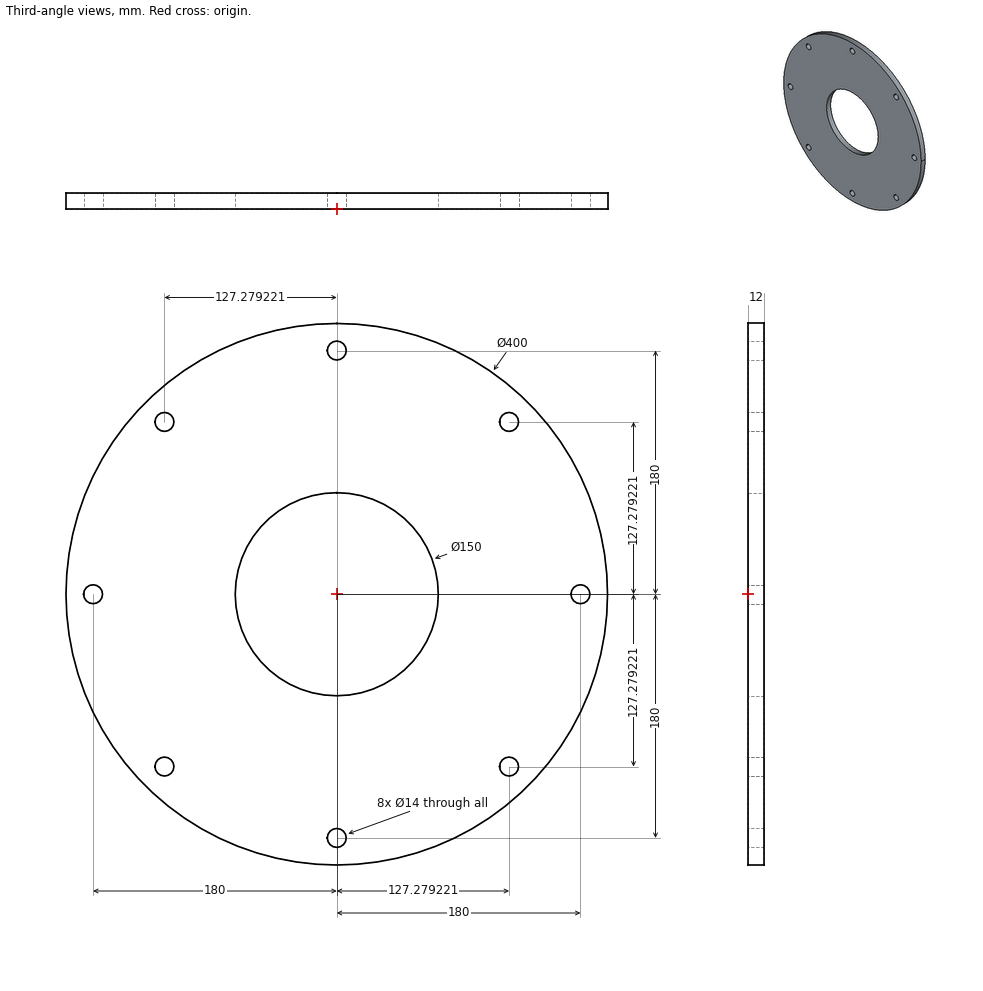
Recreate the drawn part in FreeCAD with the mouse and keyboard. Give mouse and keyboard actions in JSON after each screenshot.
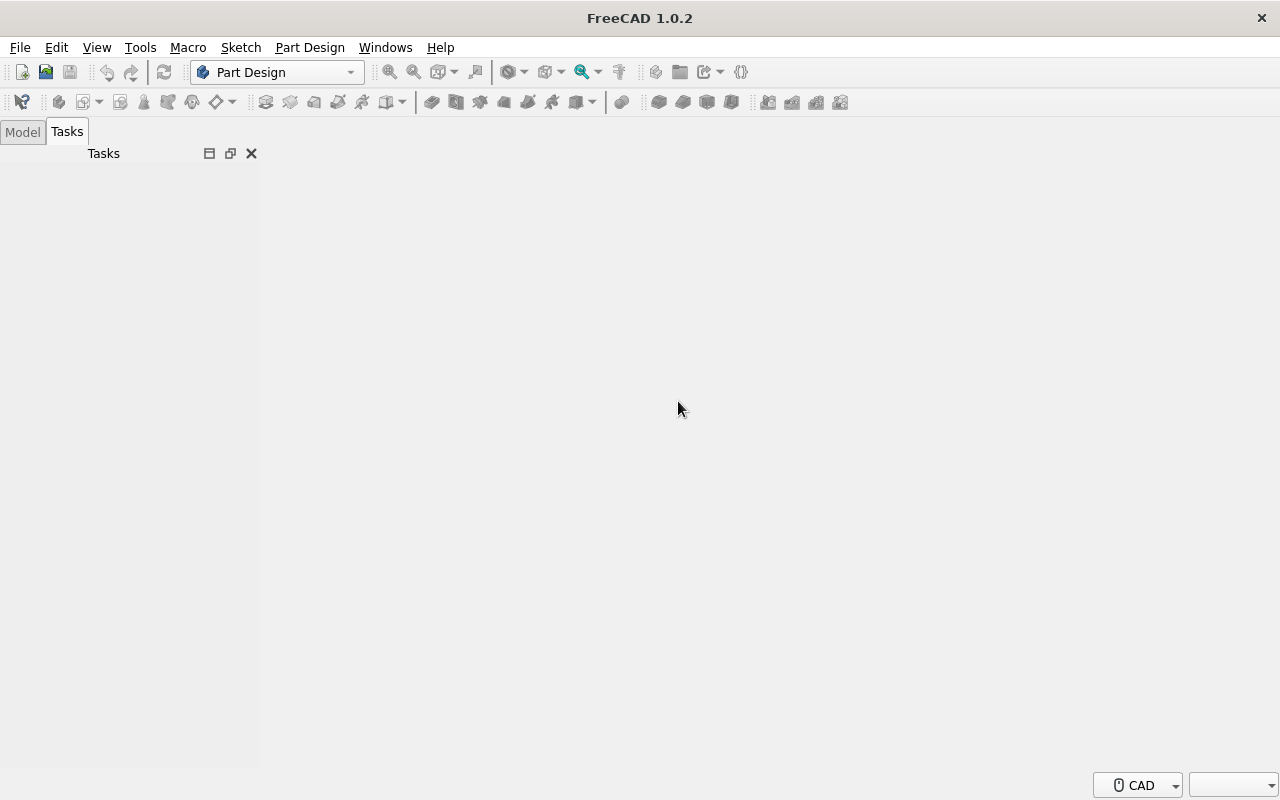
{"action": "left_click", "coordinate": [22, 72]}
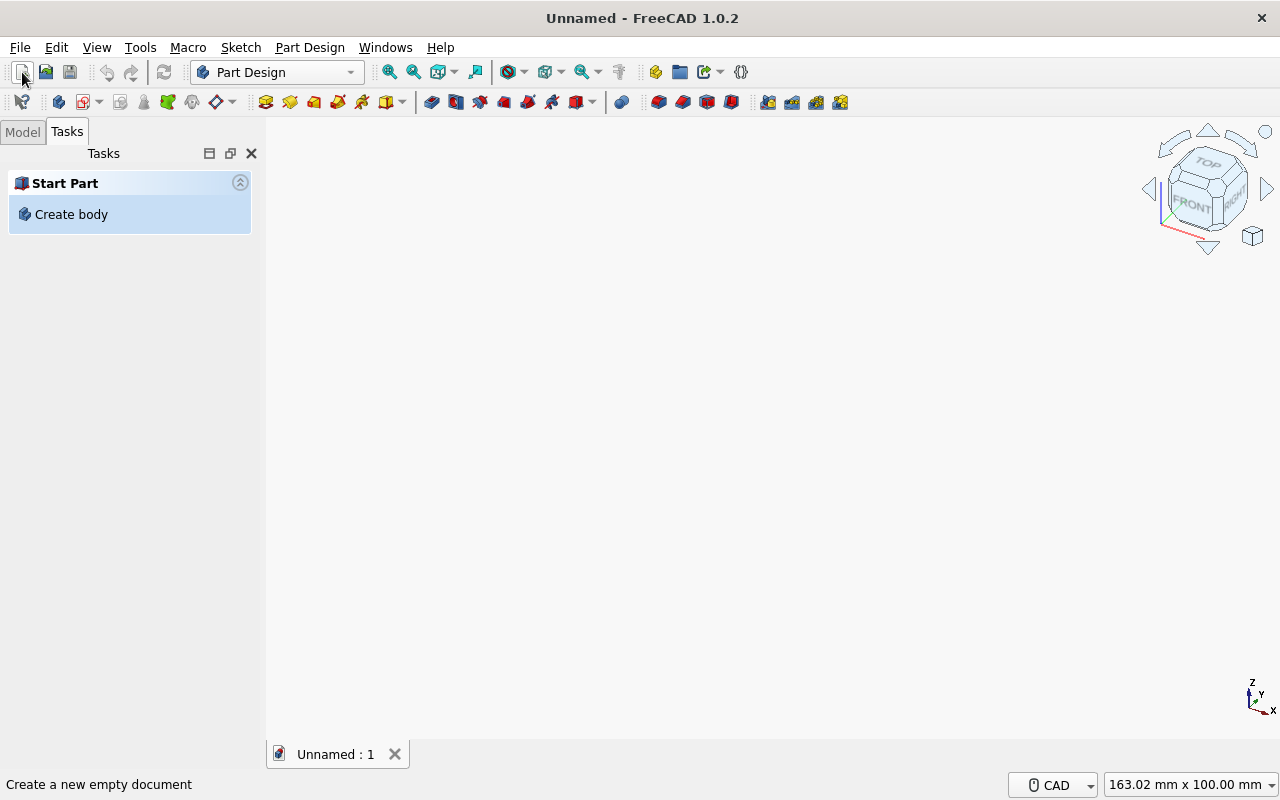
{"action": "left_click", "coordinate": [84, 102]}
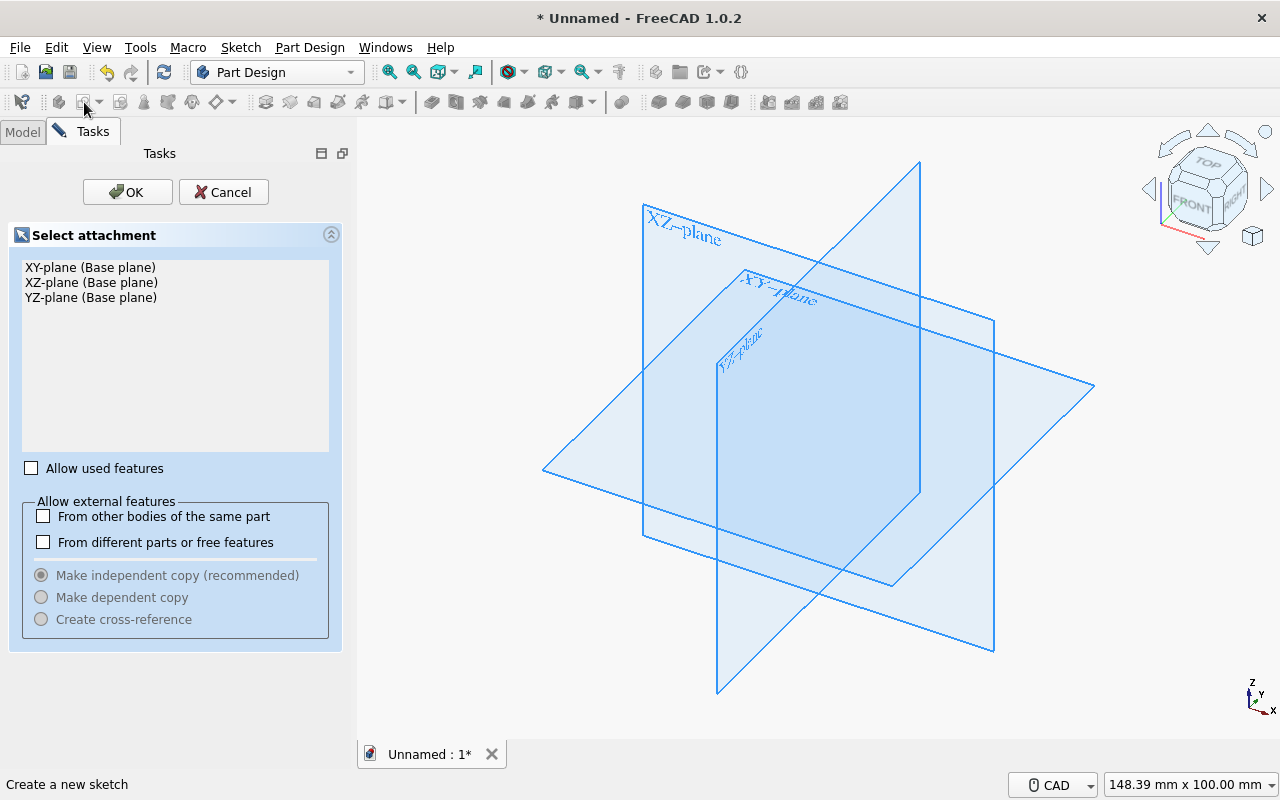
{"action": "left_click", "coordinate": [82, 282]}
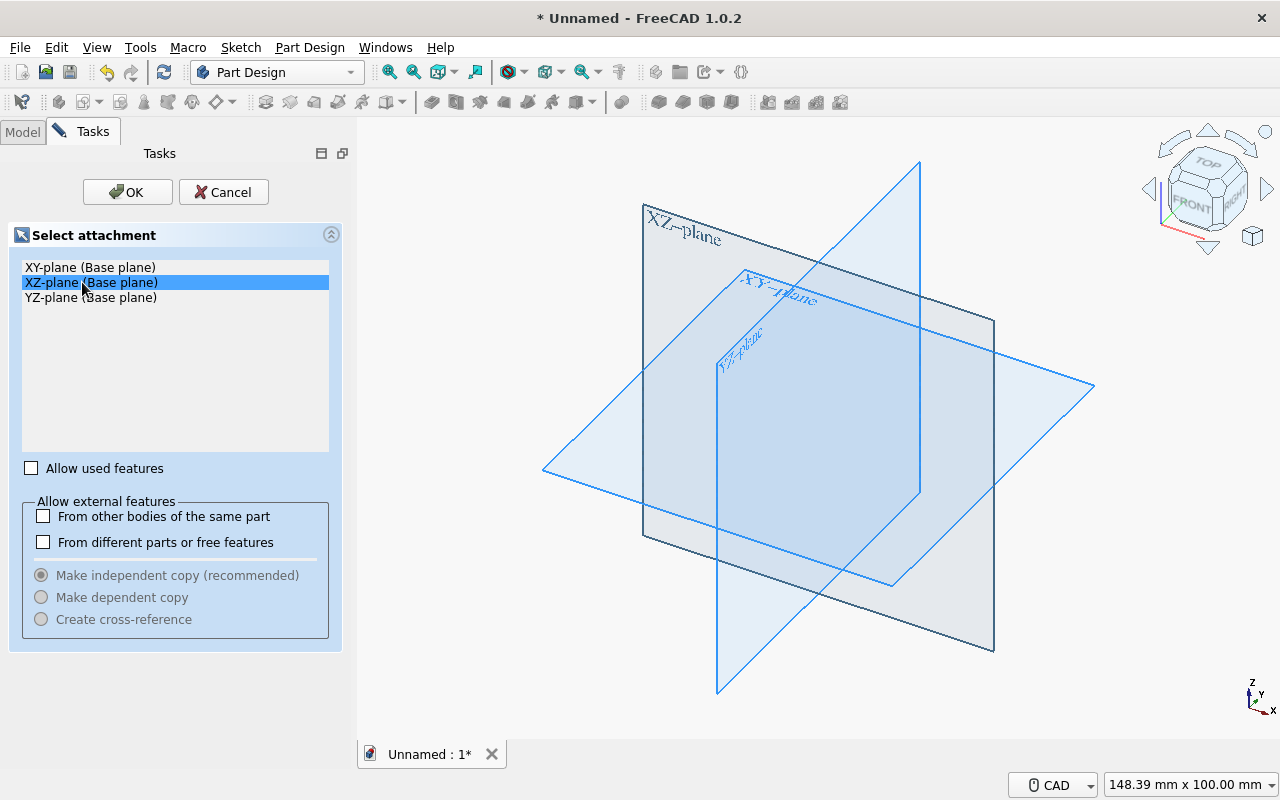
{"action": "left_click", "coordinate": [128, 192]}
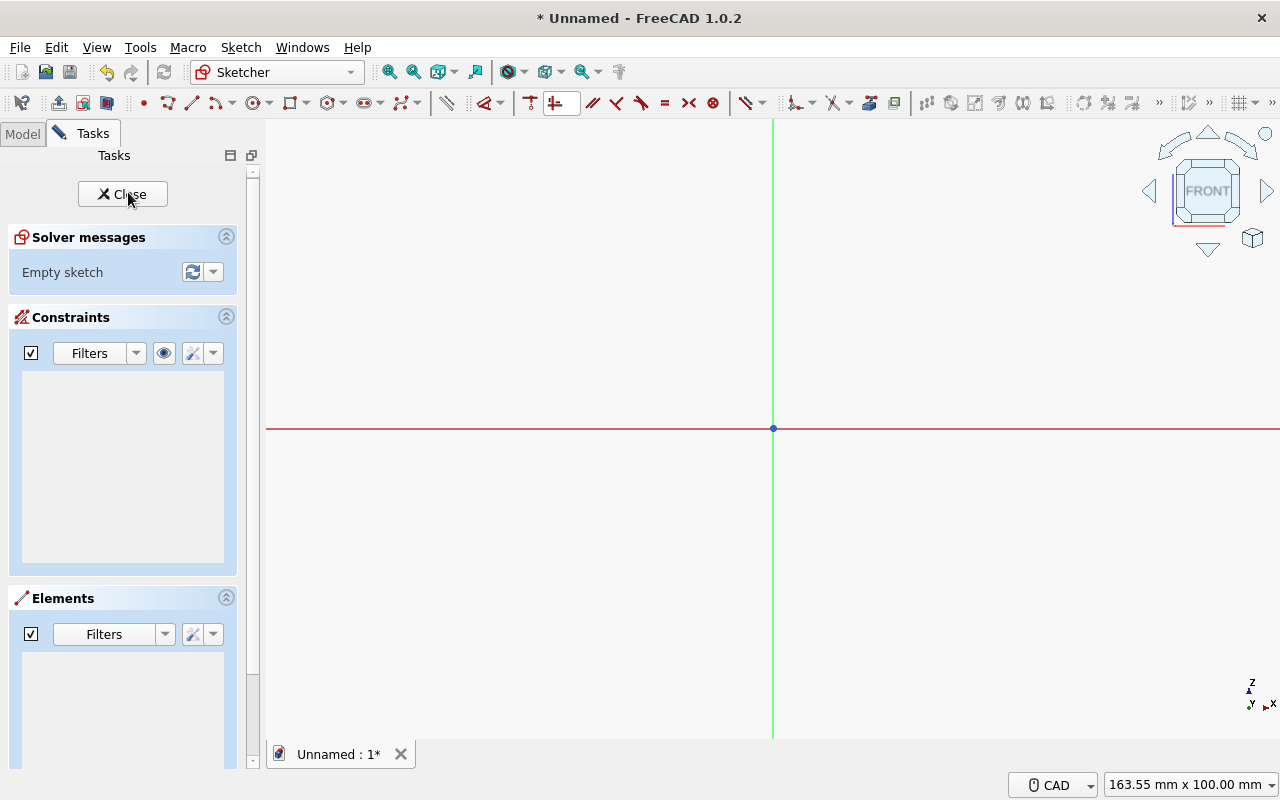
{"action": "scroll", "coordinate": [691, 429], "scroll_direction": "down", "scroll_amount": 9}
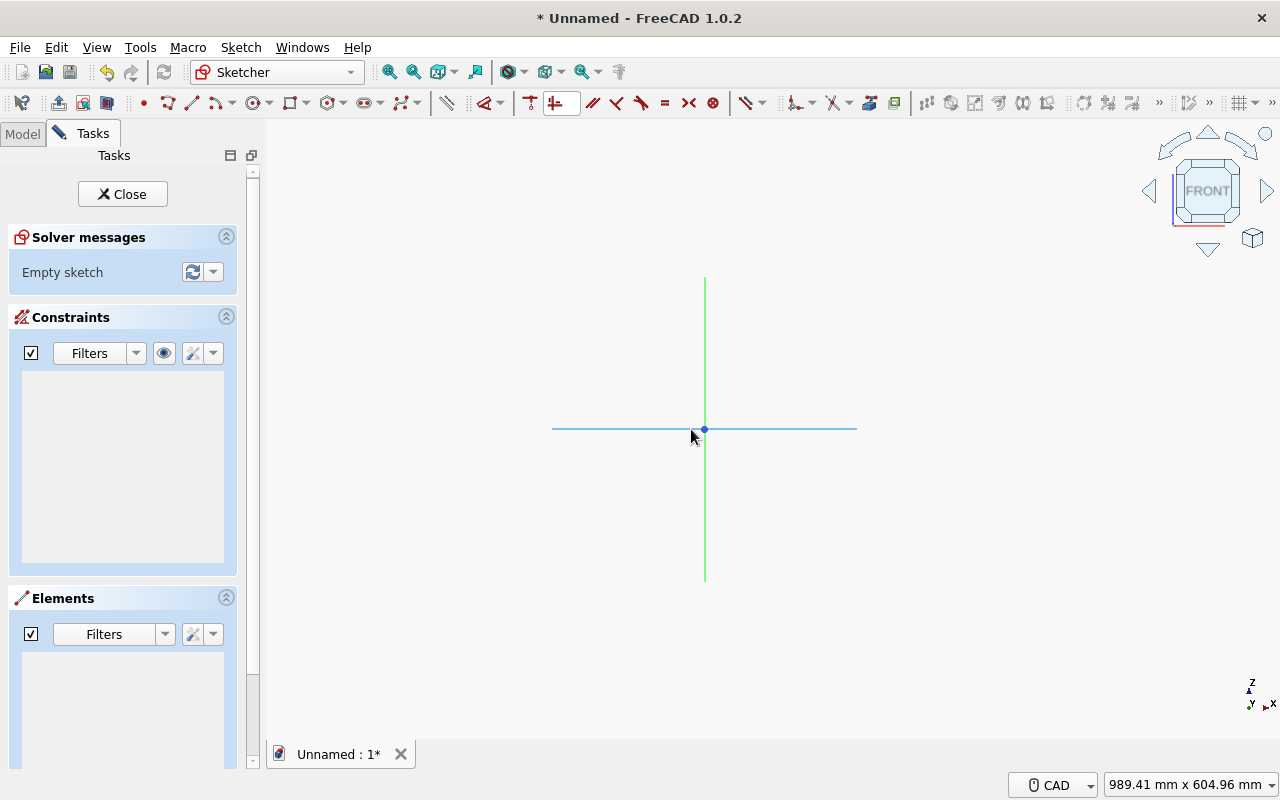
{"action": "left_click", "coordinate": [254, 104]}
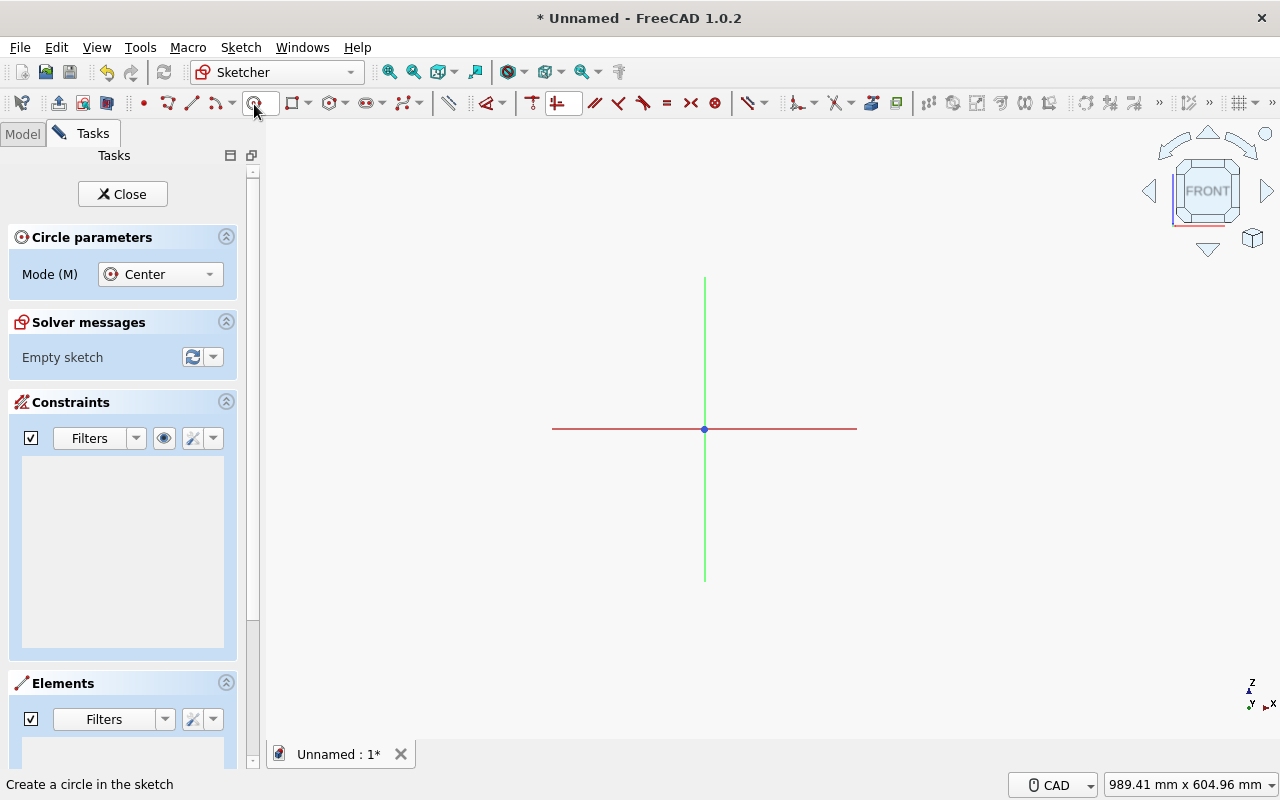
{"action": "left_click", "coordinate": [705, 429]}
{"action": "left_click", "coordinate": [850, 284]}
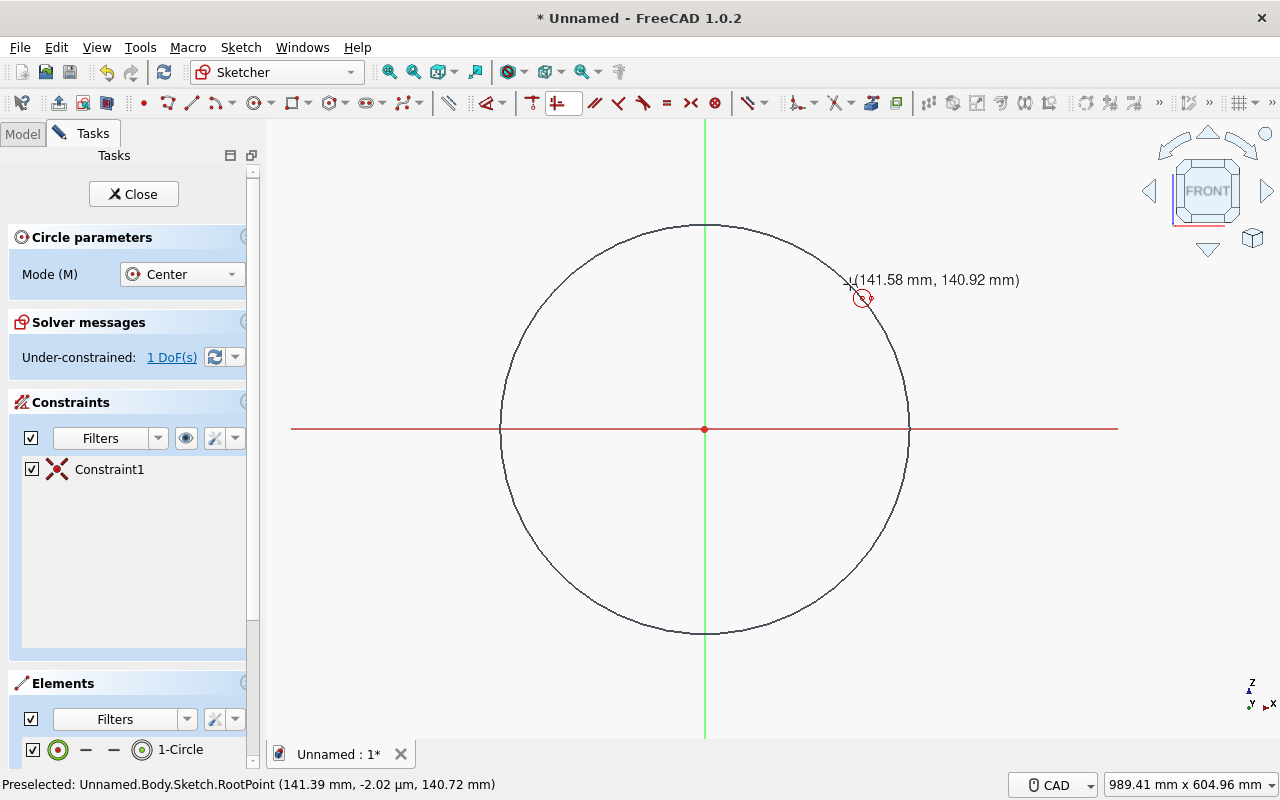
{"action": "left_click", "coordinate": [705, 429]}
{"action": "left_click", "coordinate": [759, 375]}
{"action": "key", "text": "Escape"}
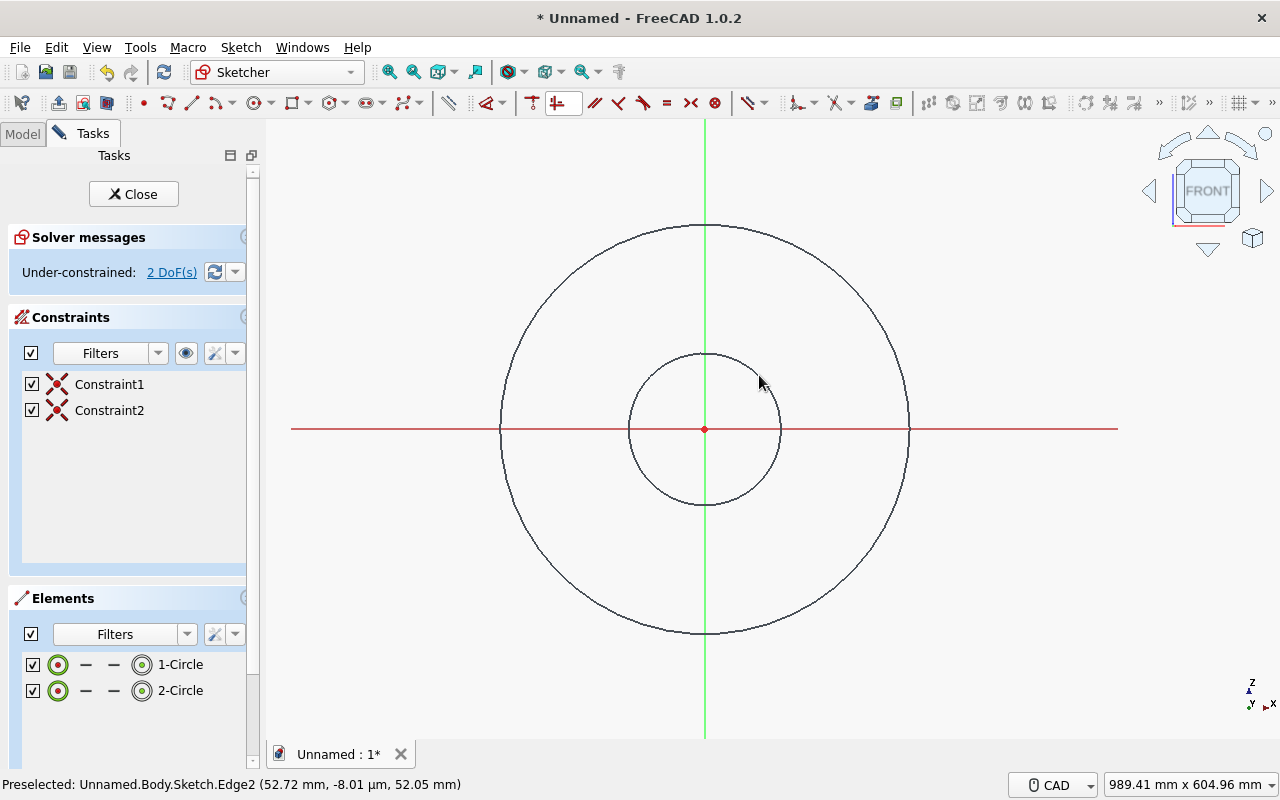
{"action": "left_click", "coordinate": [486, 104]}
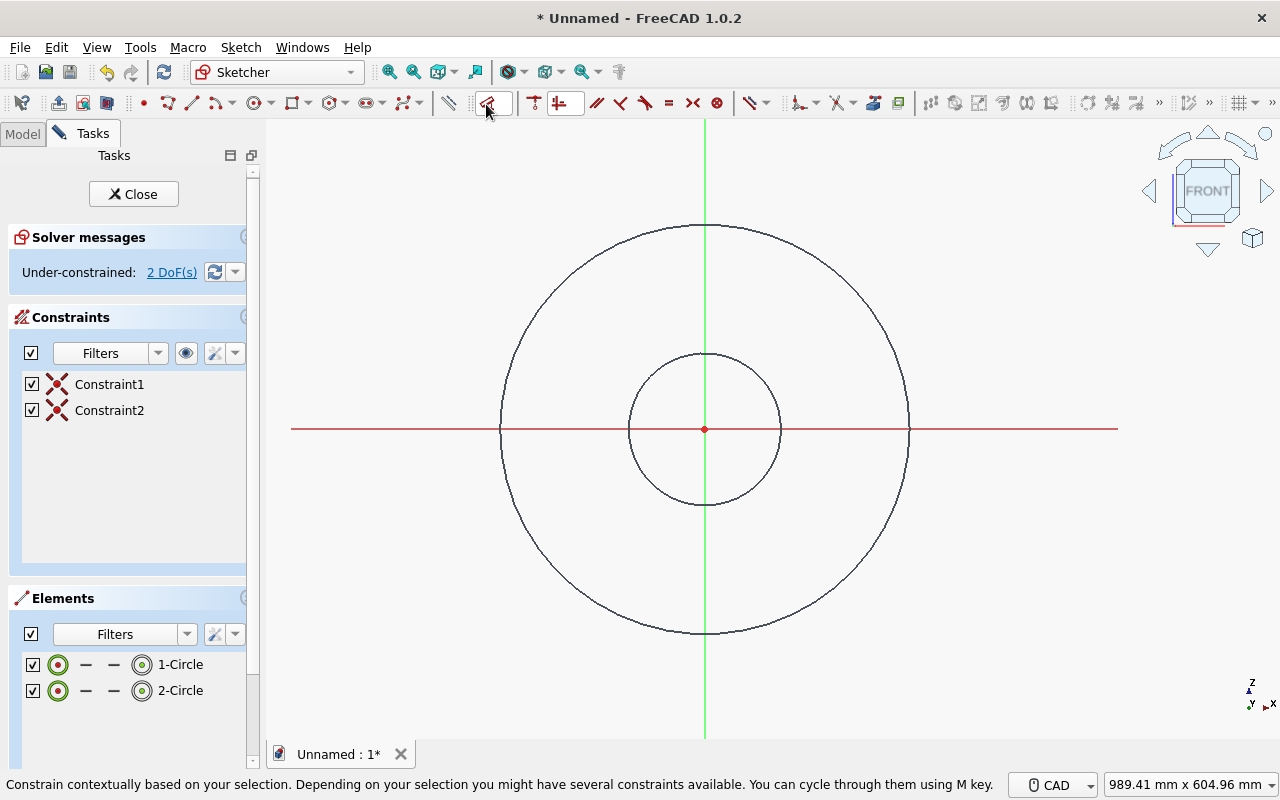
{"action": "left_click", "coordinate": [849, 284]}
{"action": "left_click", "coordinate": [872, 261]}